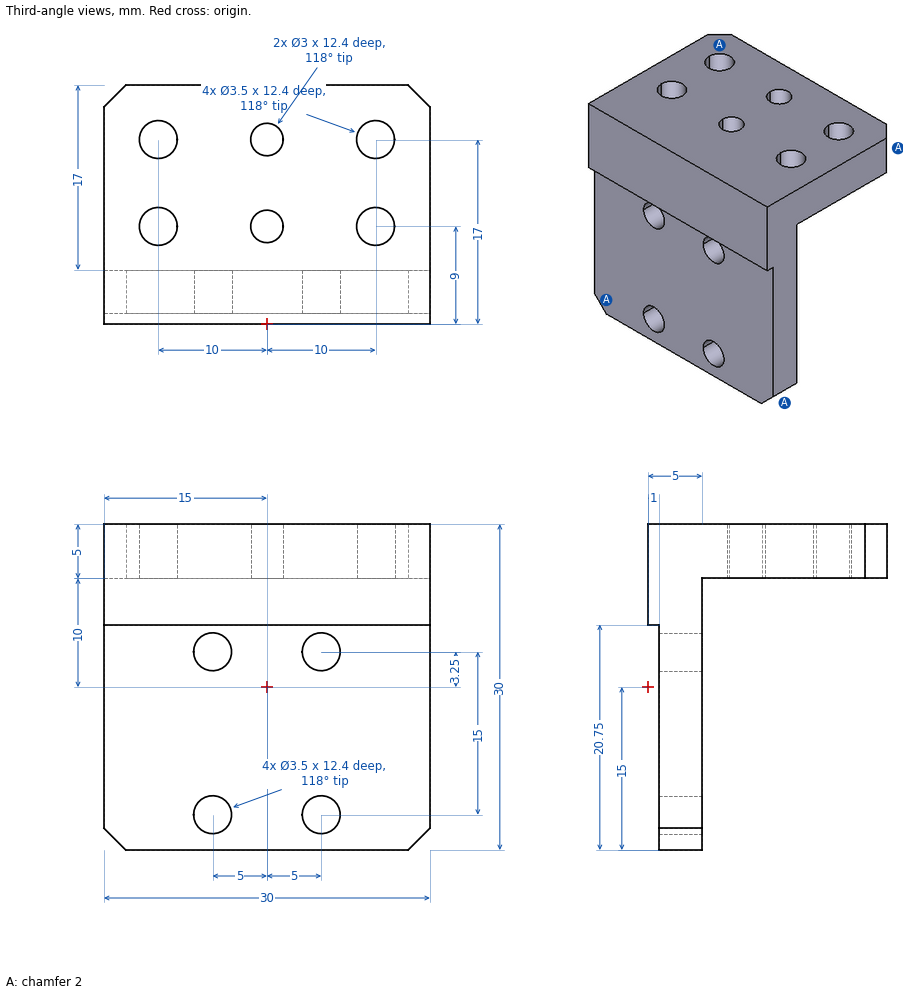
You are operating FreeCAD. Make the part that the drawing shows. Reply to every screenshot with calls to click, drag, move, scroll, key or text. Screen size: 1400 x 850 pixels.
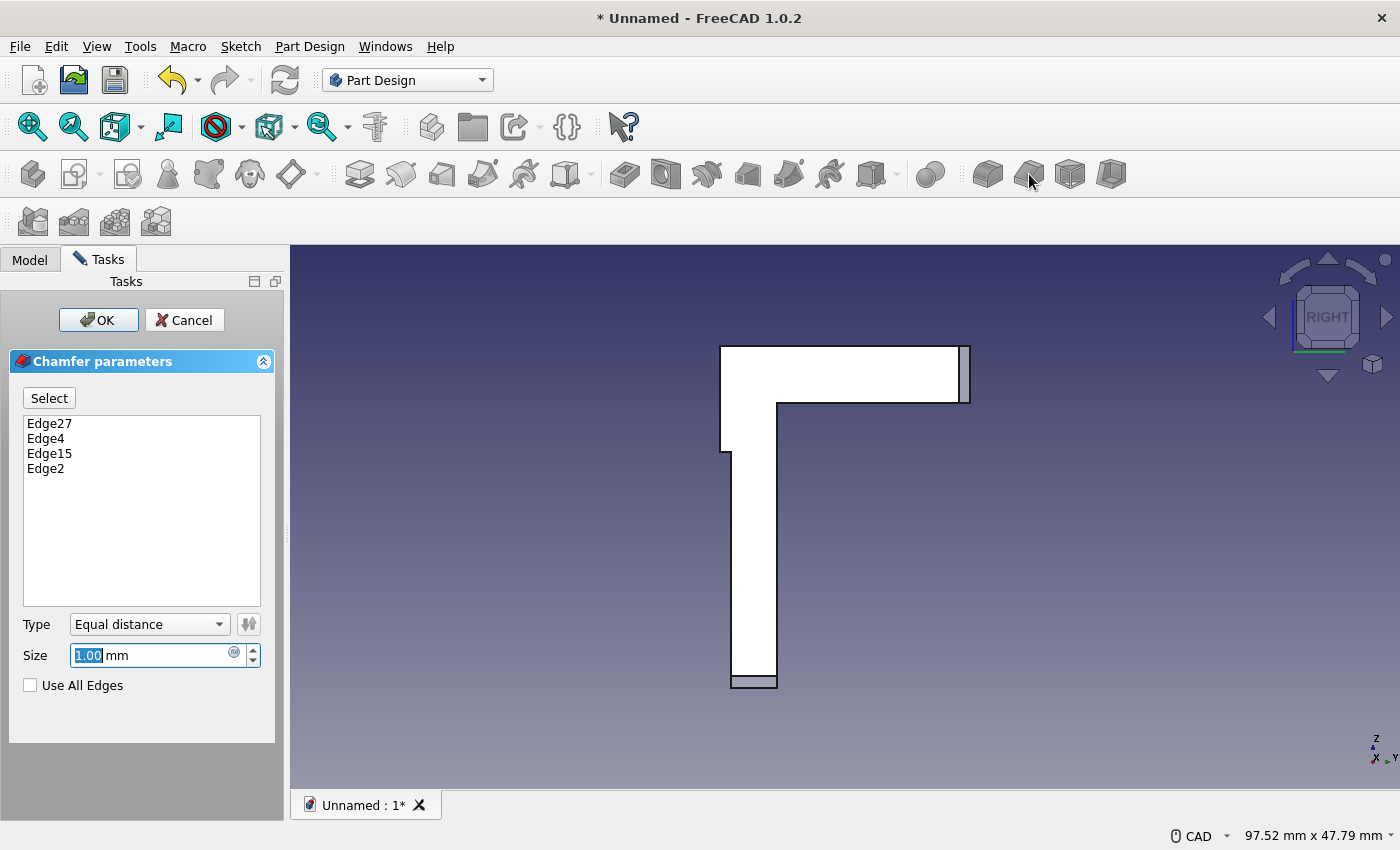
text(2)
key(Tab)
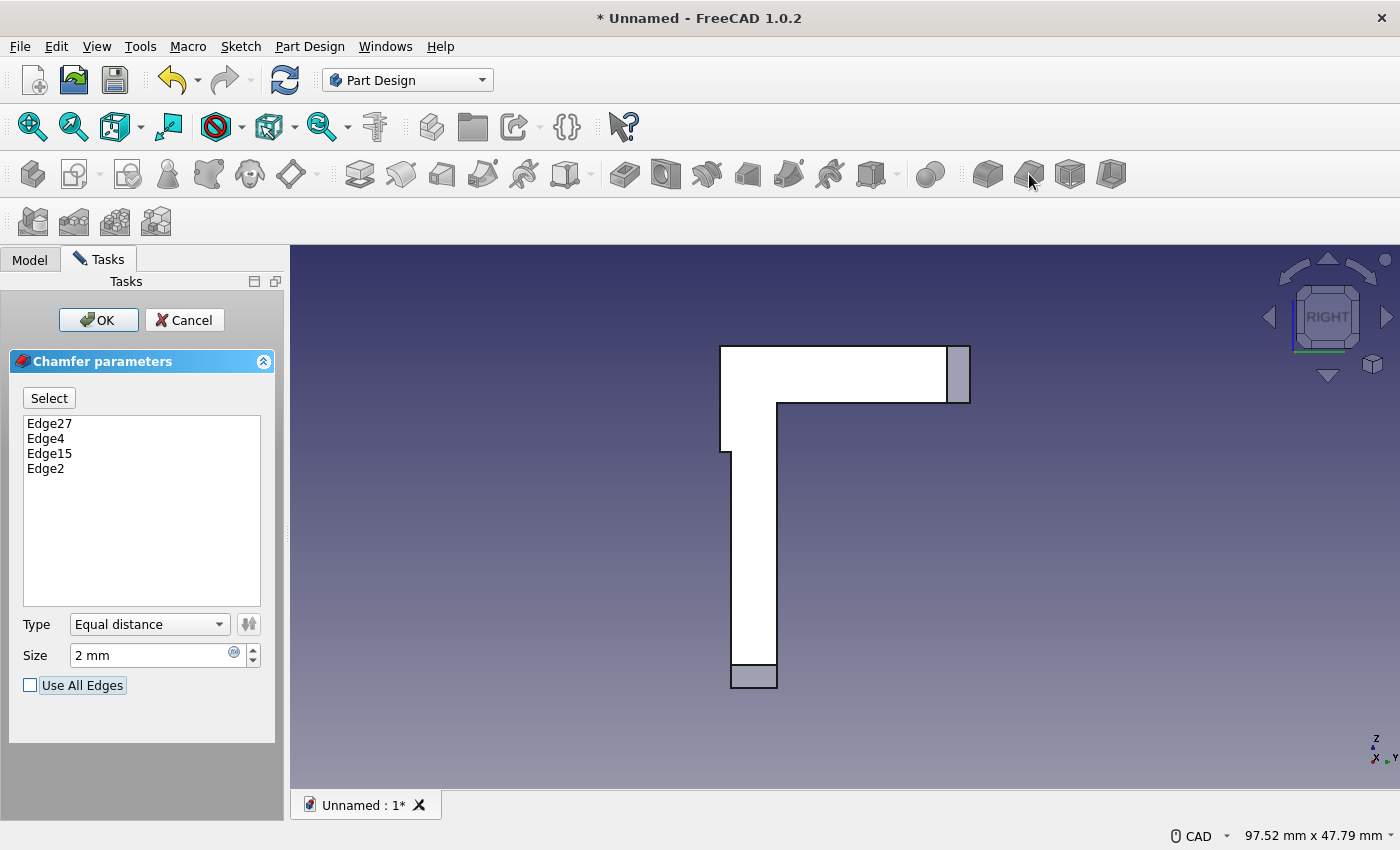
click(99, 320)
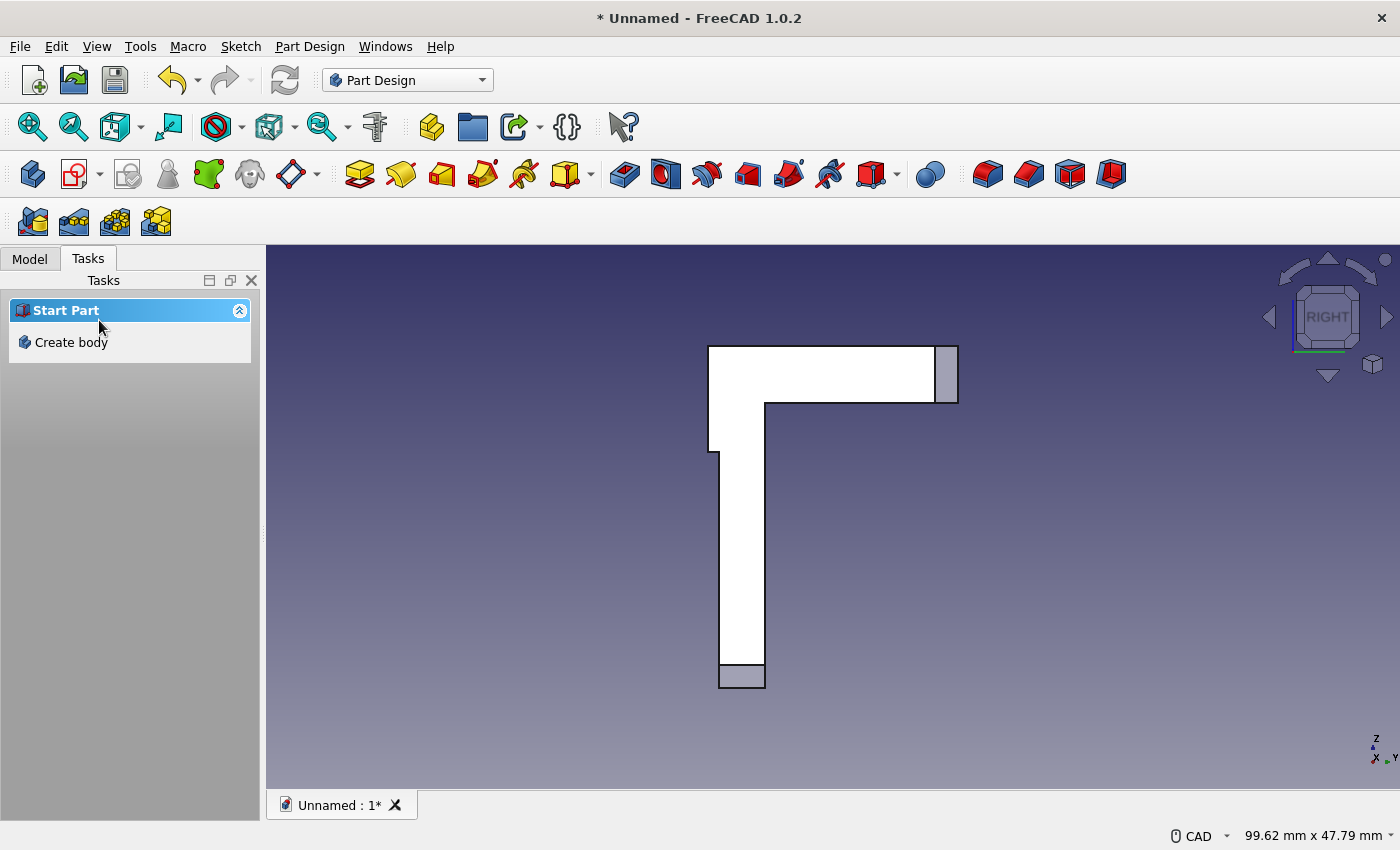
key(5)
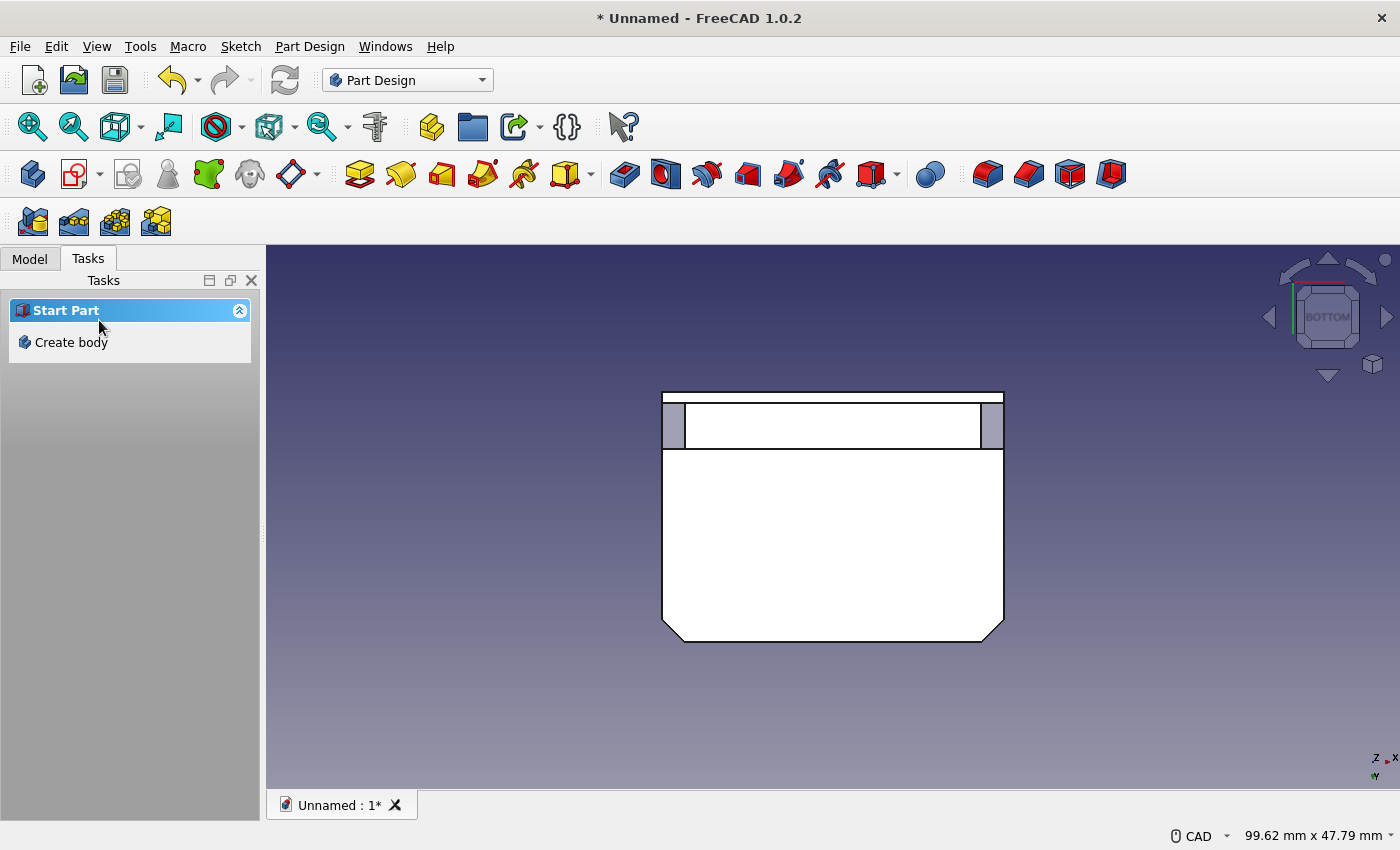
click(882, 544)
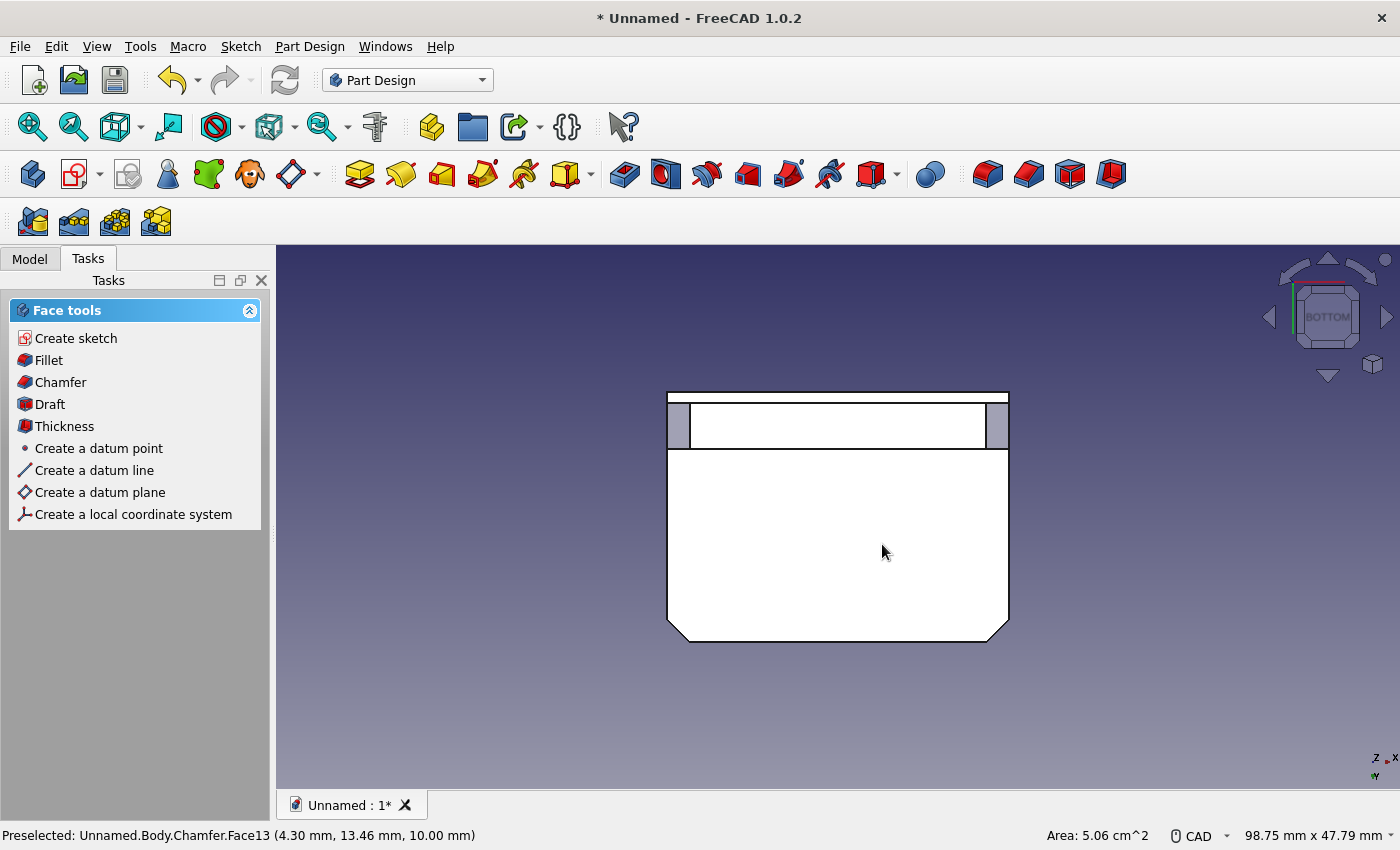
click(74, 174)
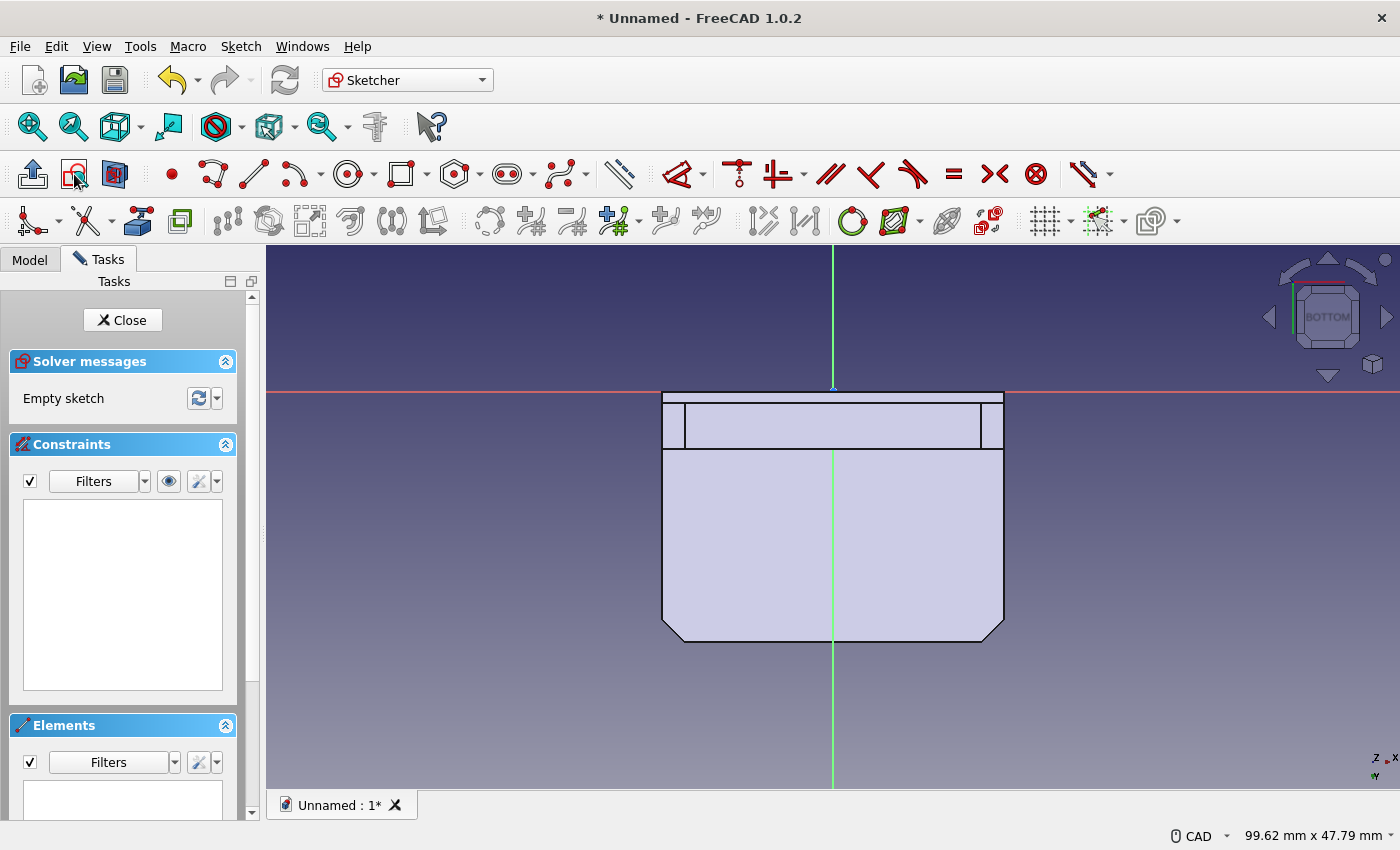
key(q)
key(s)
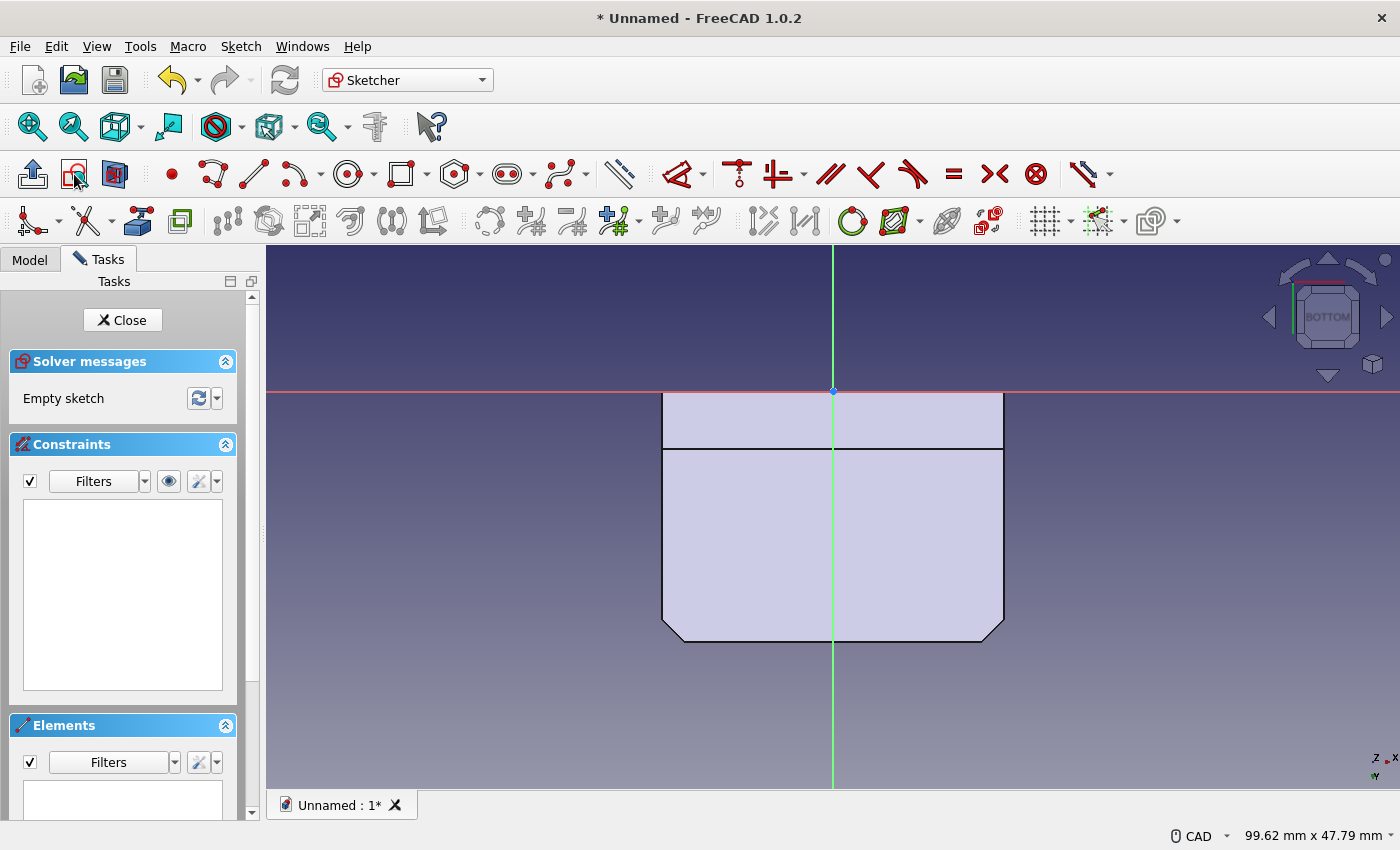
scroll(972, 461, up, 2)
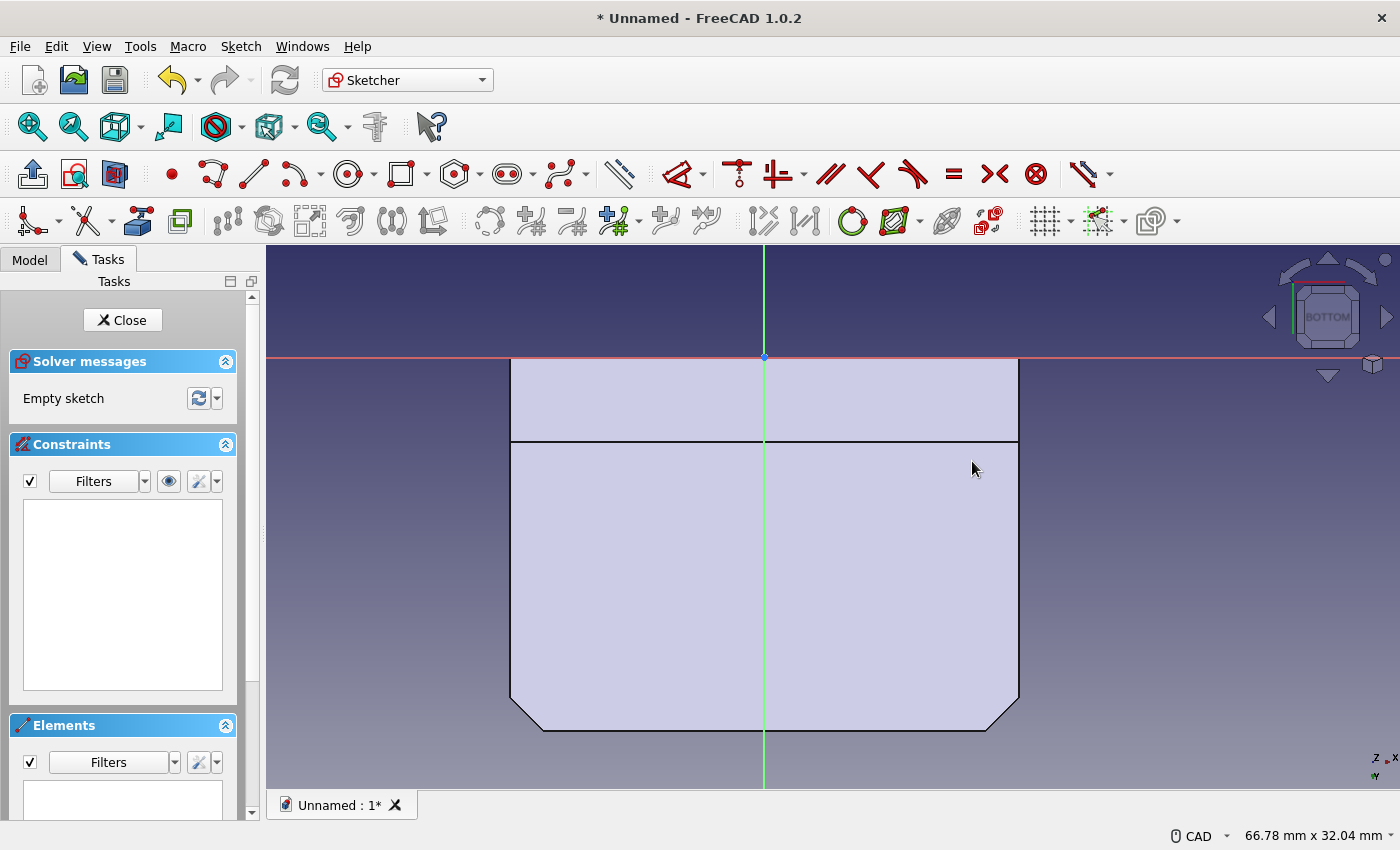
click(348, 174)